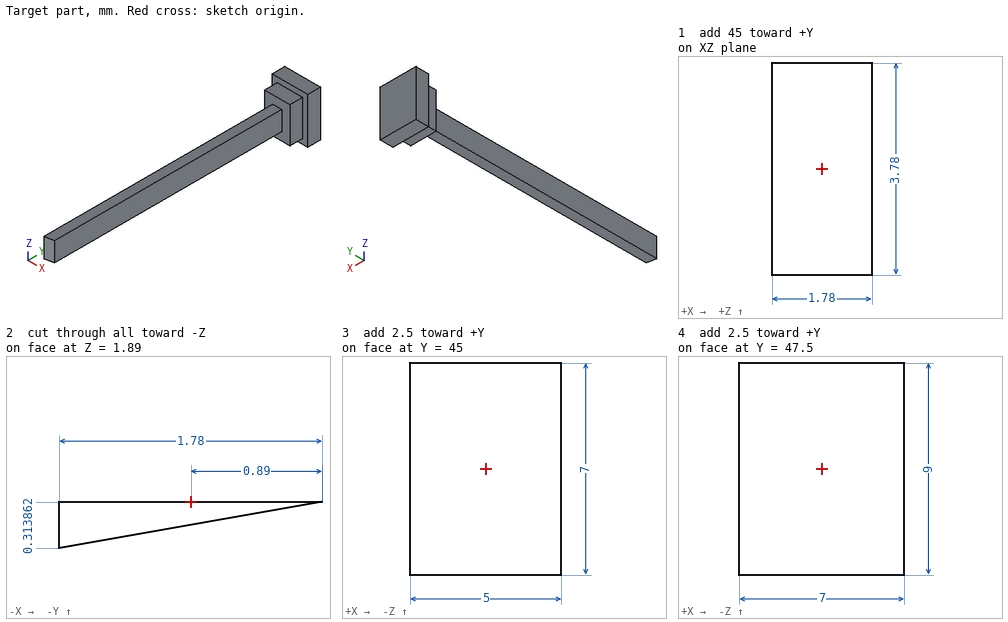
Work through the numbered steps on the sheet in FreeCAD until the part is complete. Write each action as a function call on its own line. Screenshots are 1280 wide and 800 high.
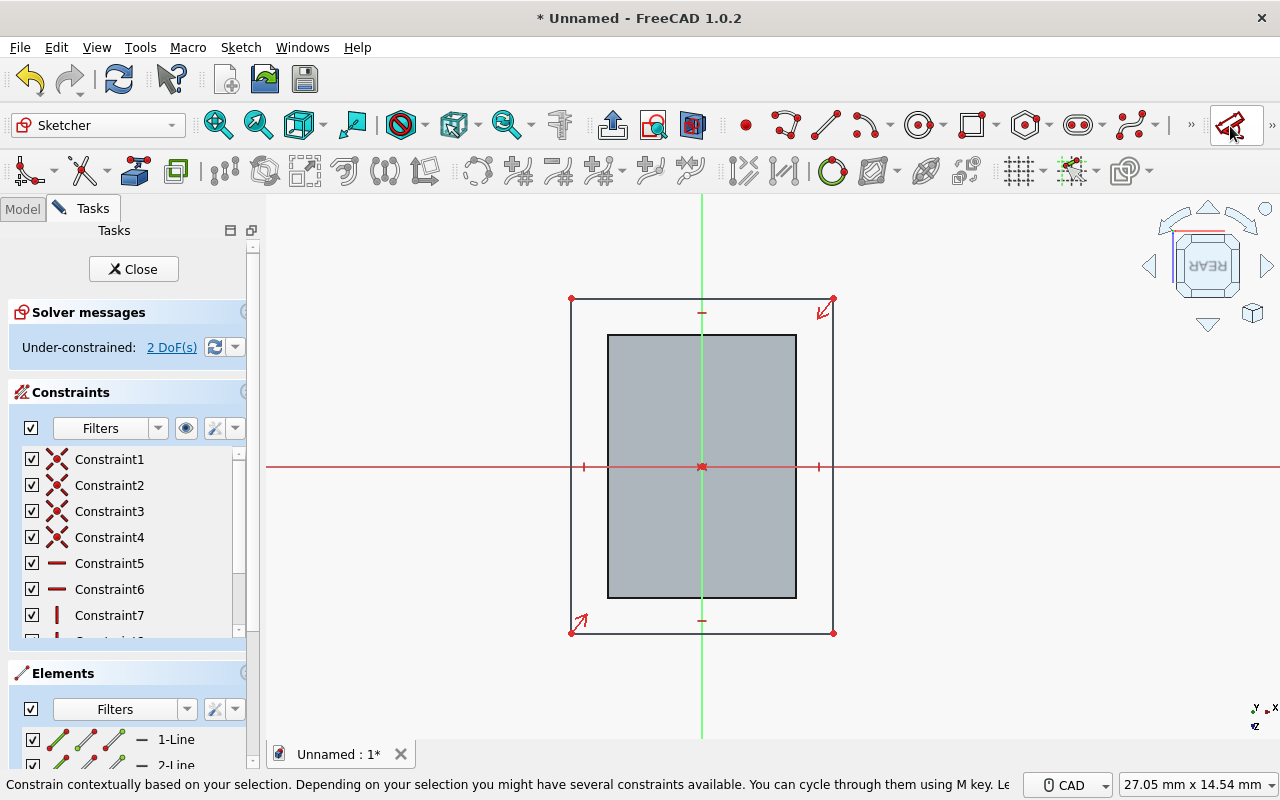
click(650, 634)
click(642, 668)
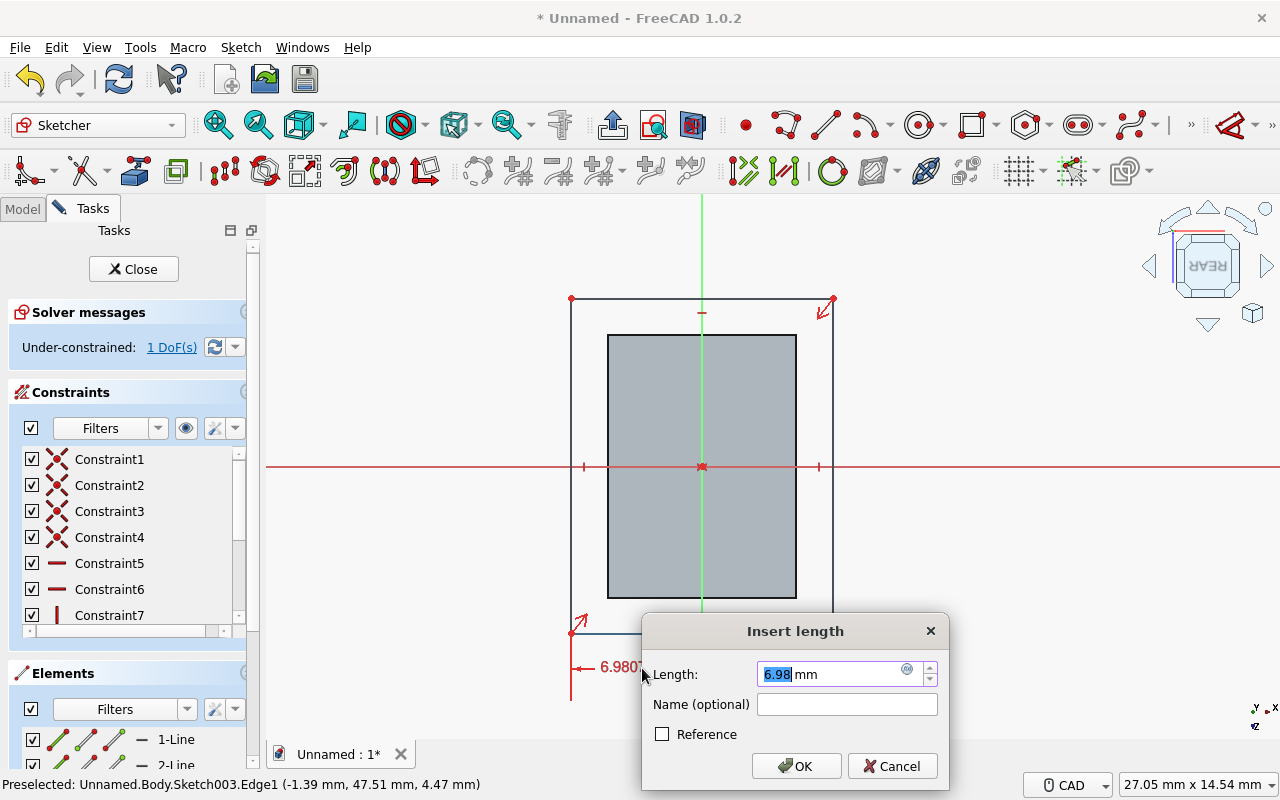
text(7)
key(Return)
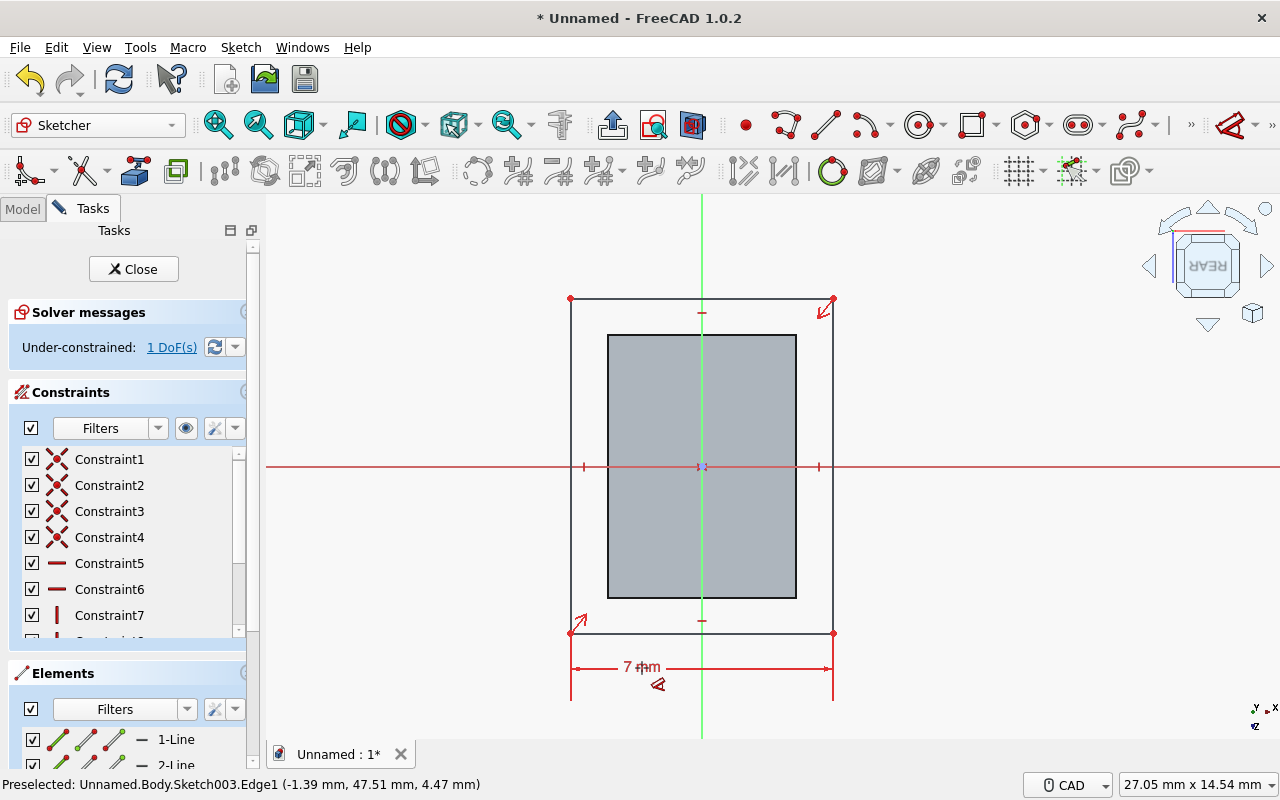
click(833, 533)
click(867, 389)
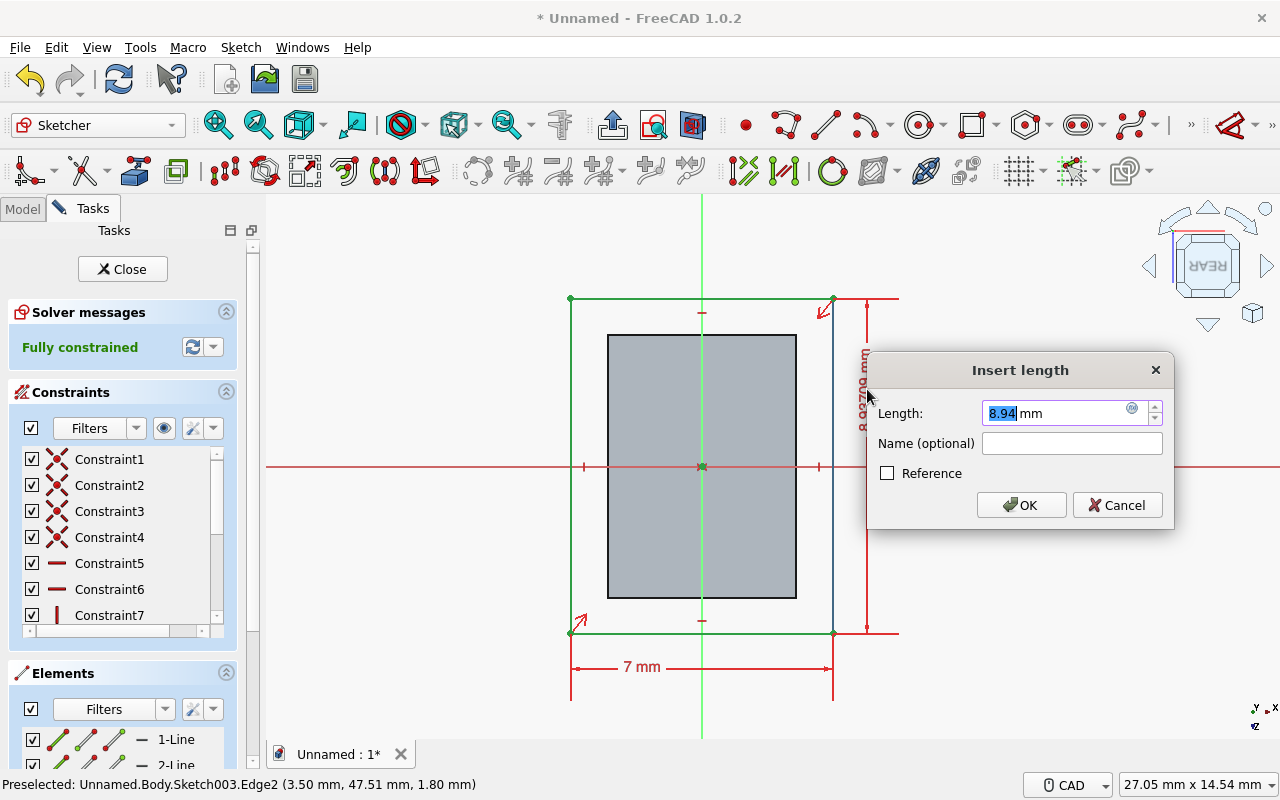
text(9)
key(Return)
key(Escape)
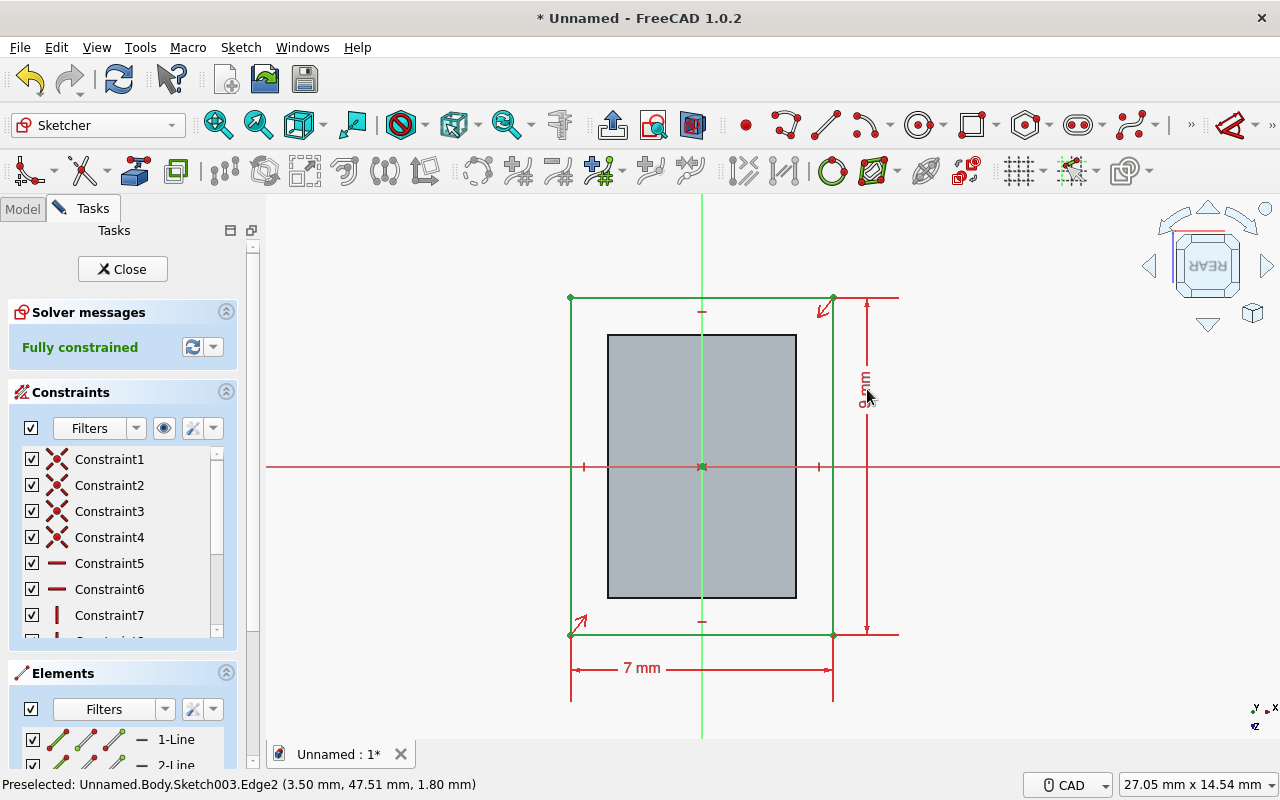
click(123, 269)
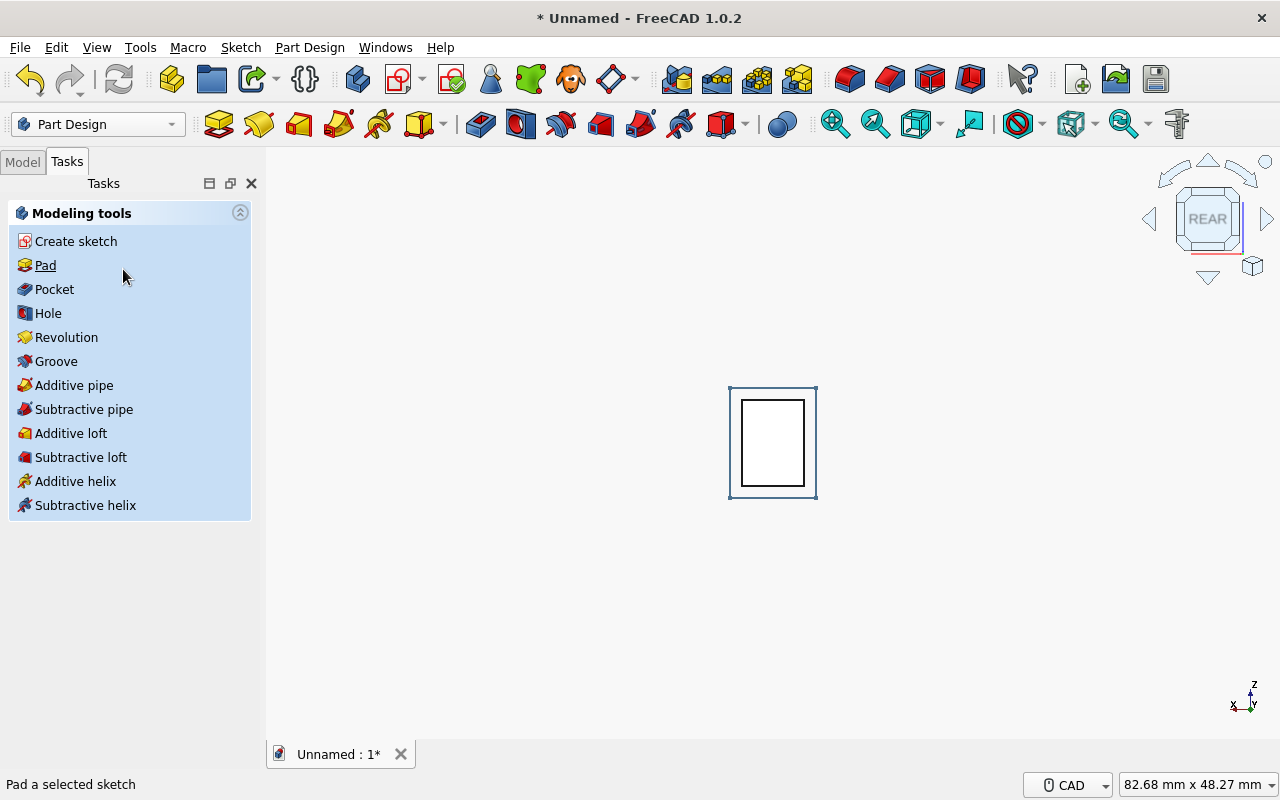
click(220, 124)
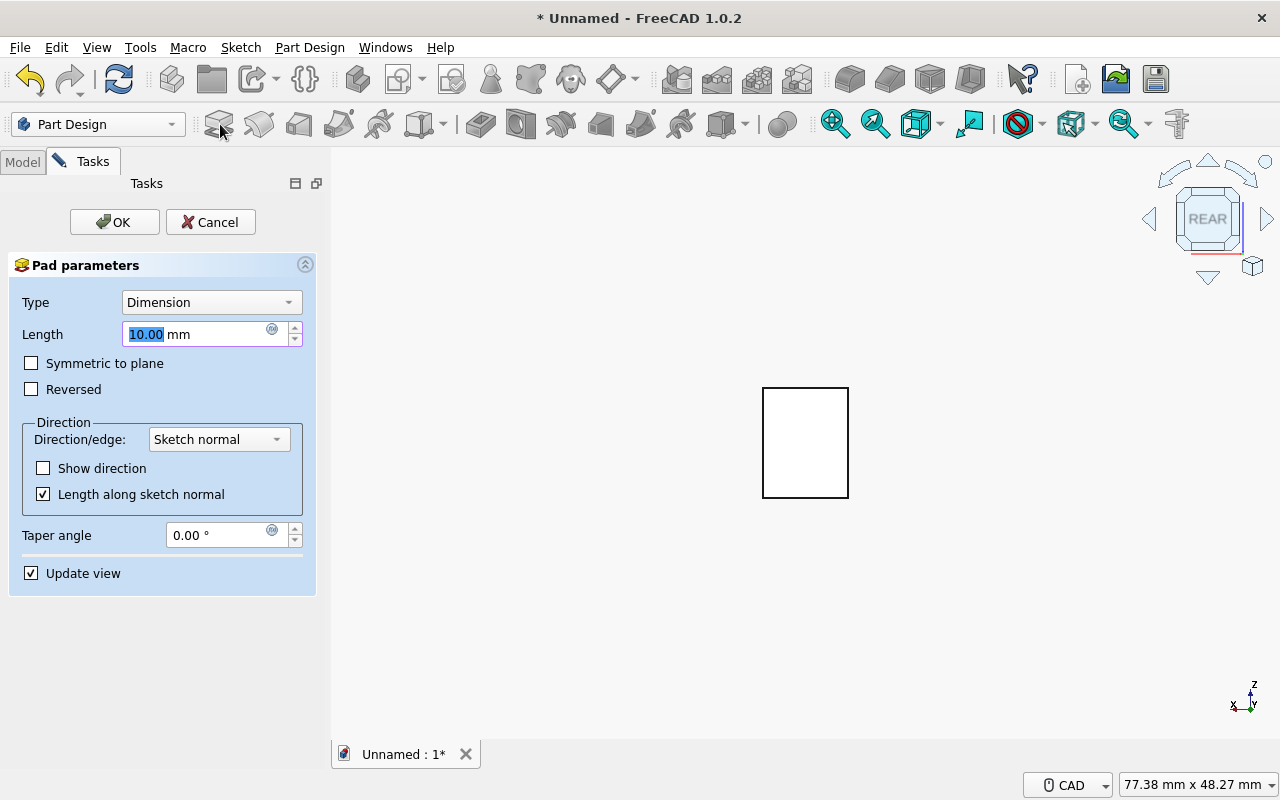
text(2.5)
key(Tab)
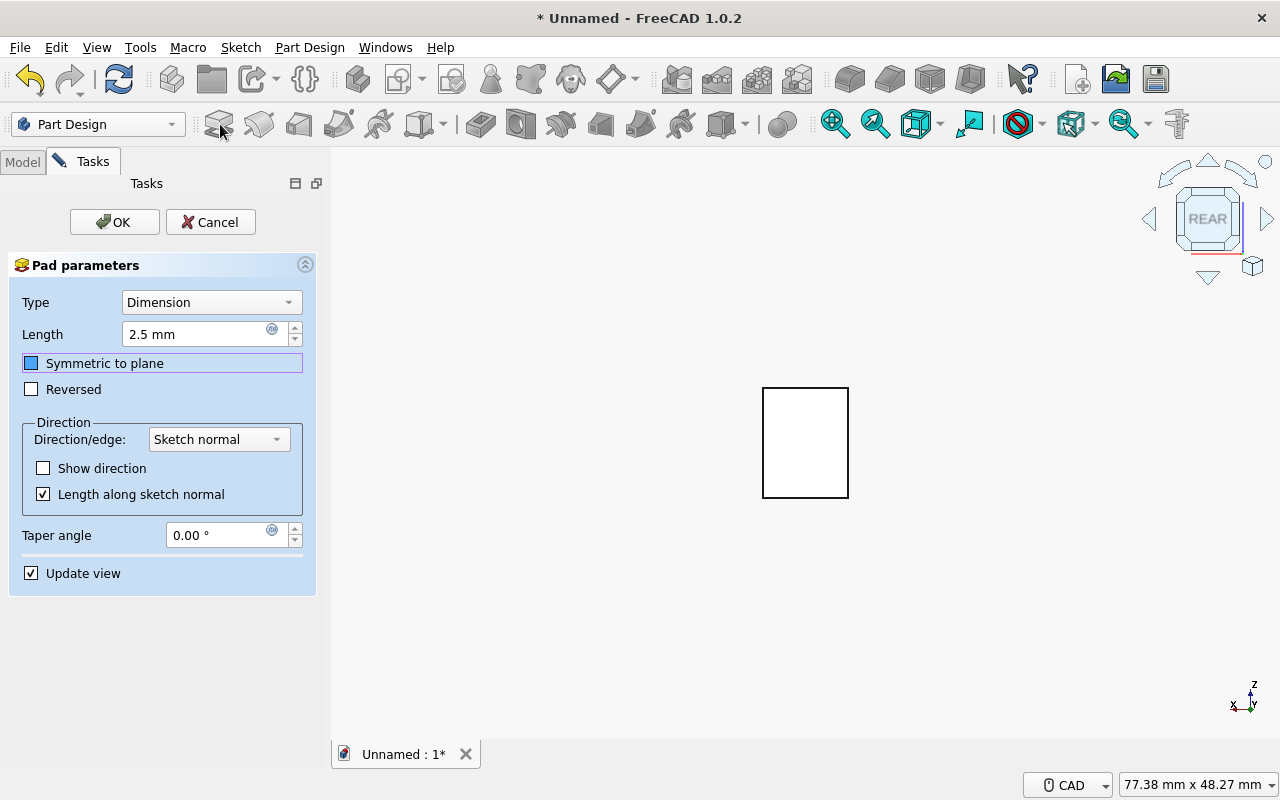
click(115, 222)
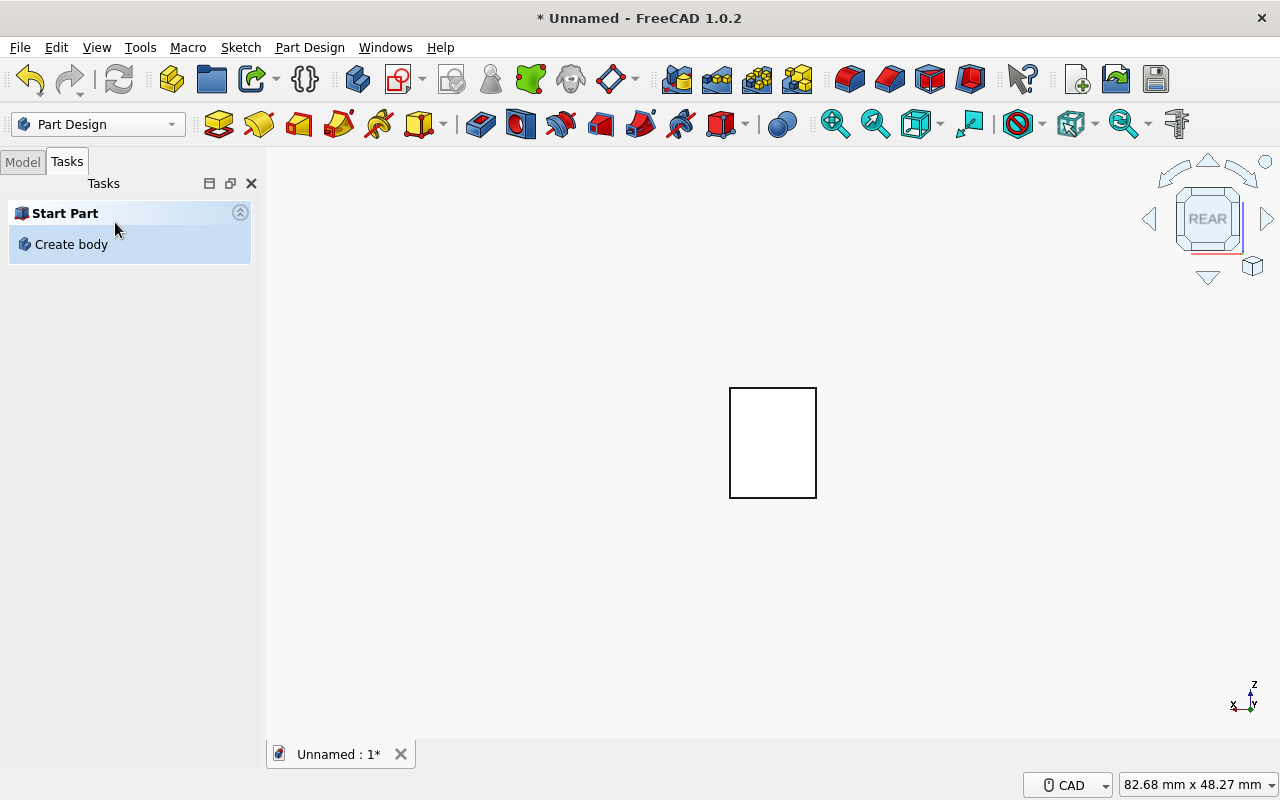
key(0)